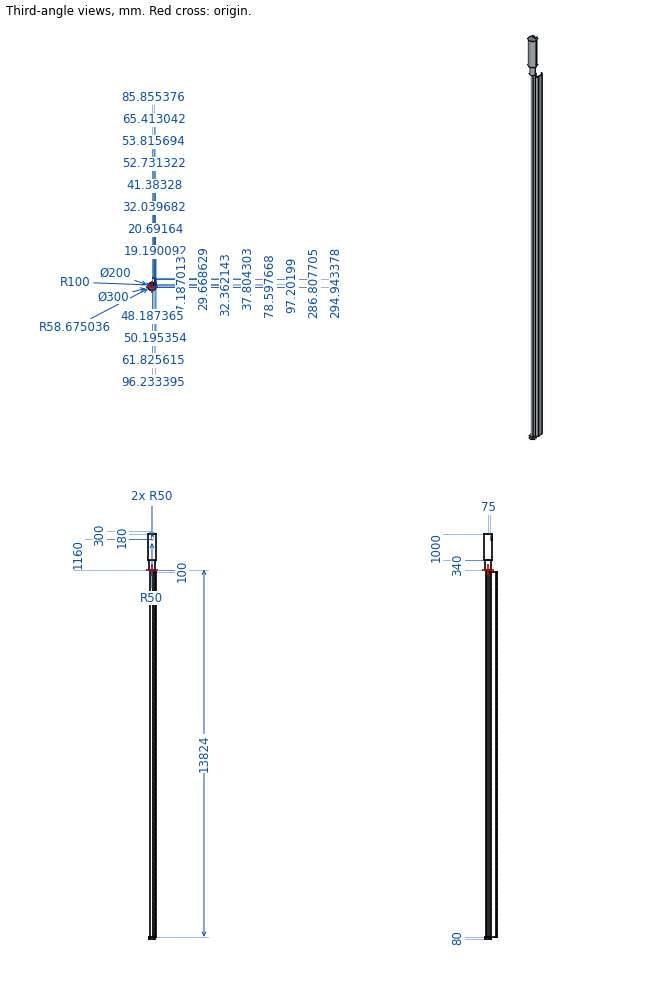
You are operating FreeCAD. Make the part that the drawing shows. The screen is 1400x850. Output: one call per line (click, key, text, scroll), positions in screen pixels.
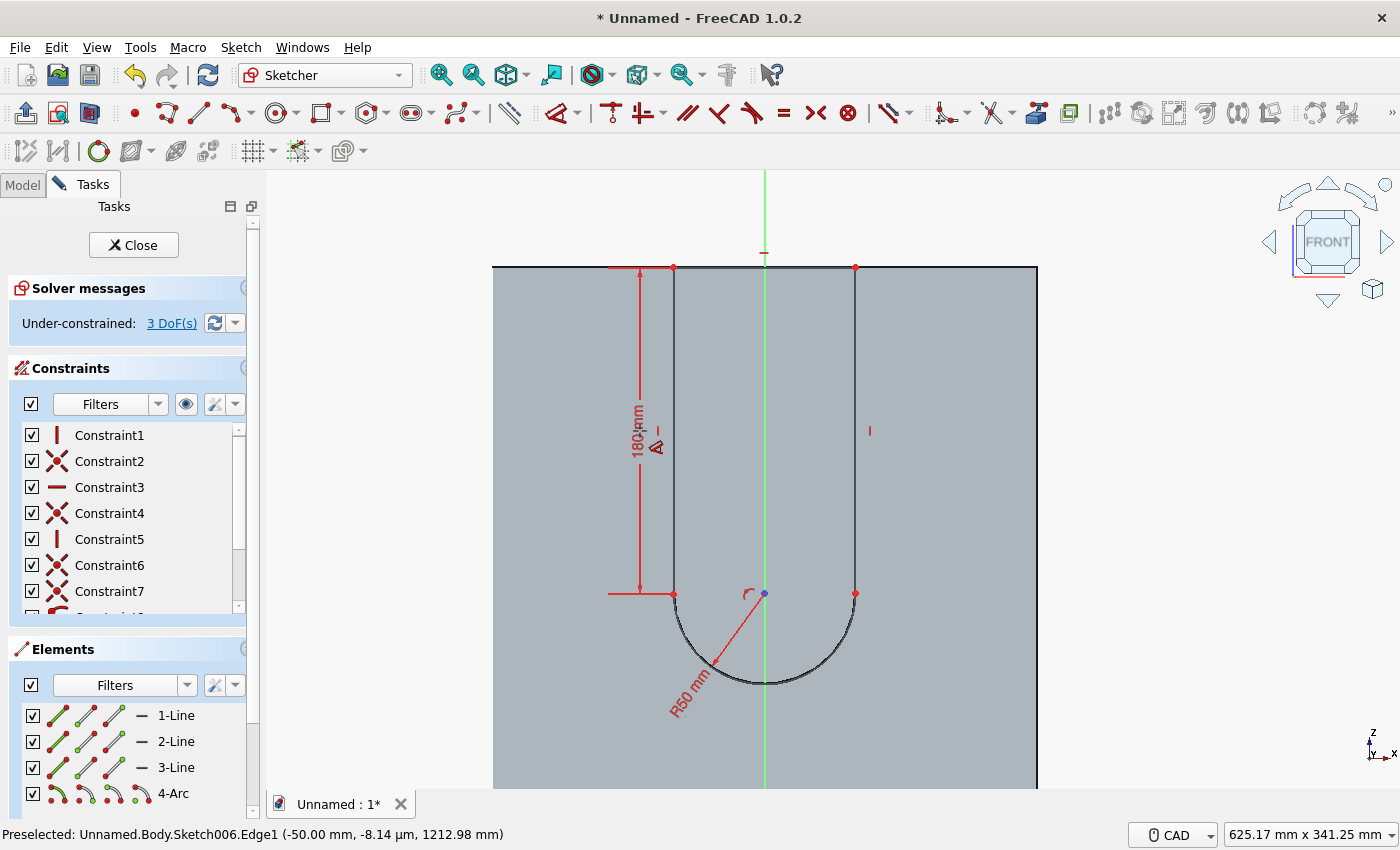
click(855, 366)
click(889, 431)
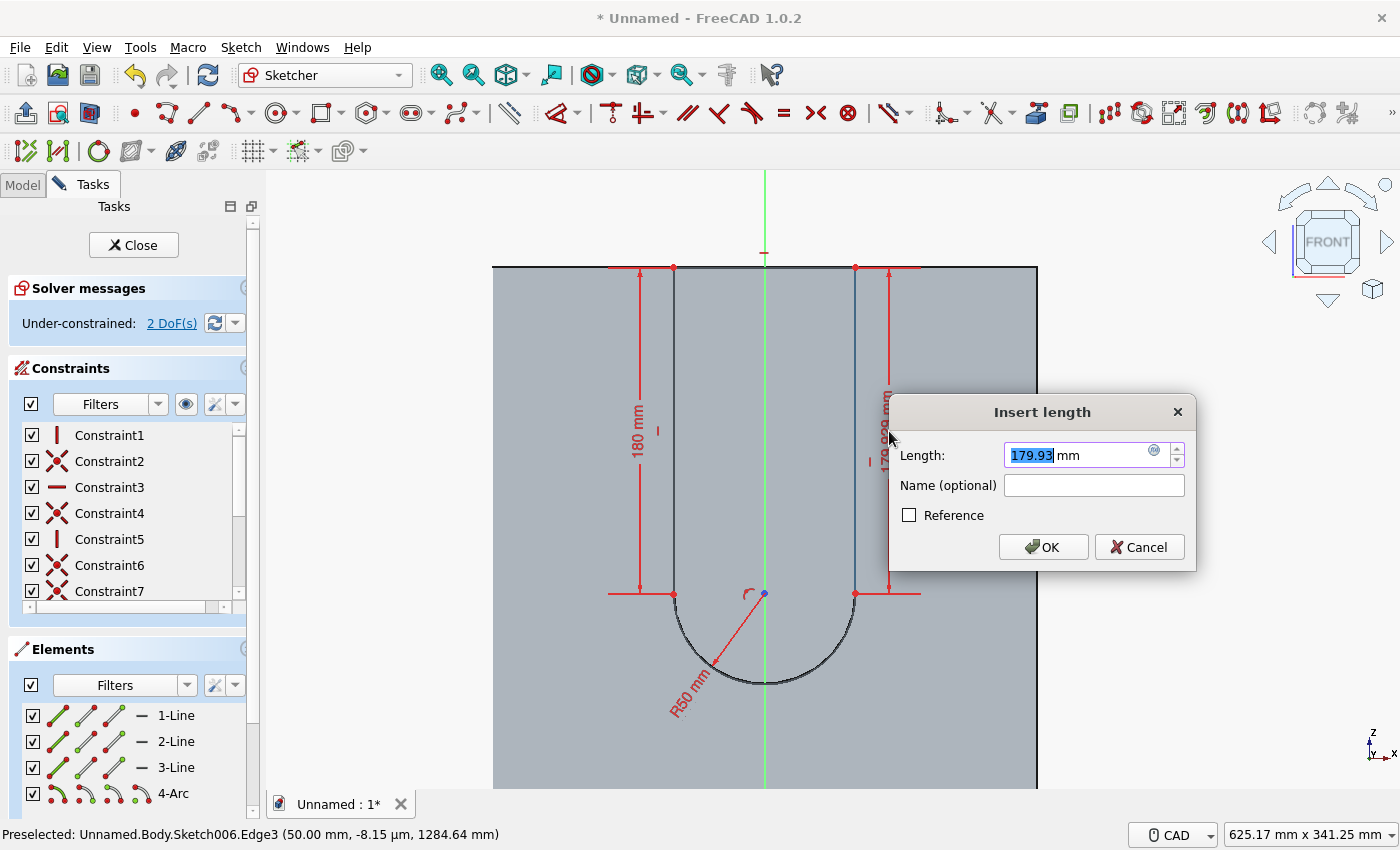
text(180)
key(Return)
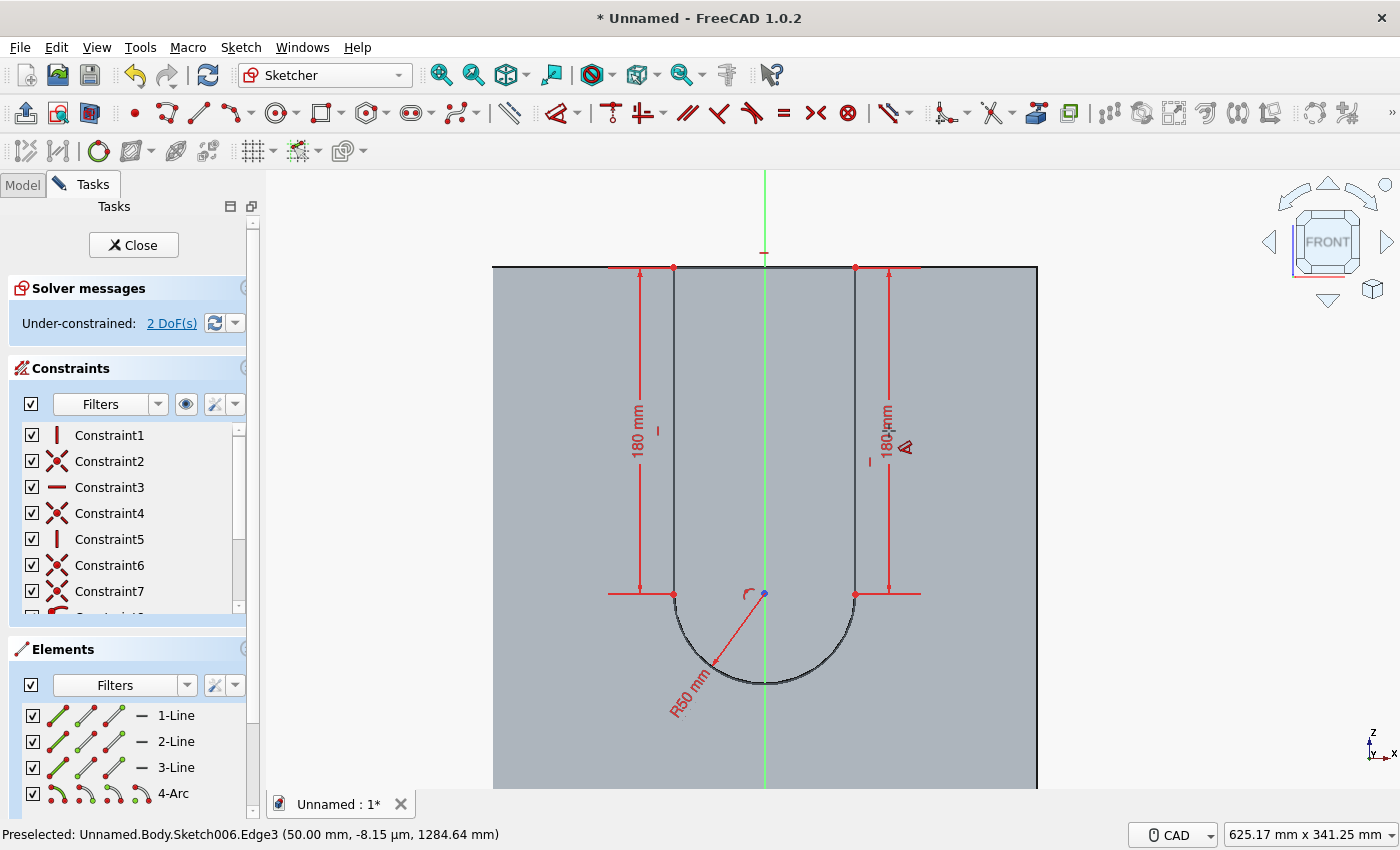
click(674, 594)
click(640, 639)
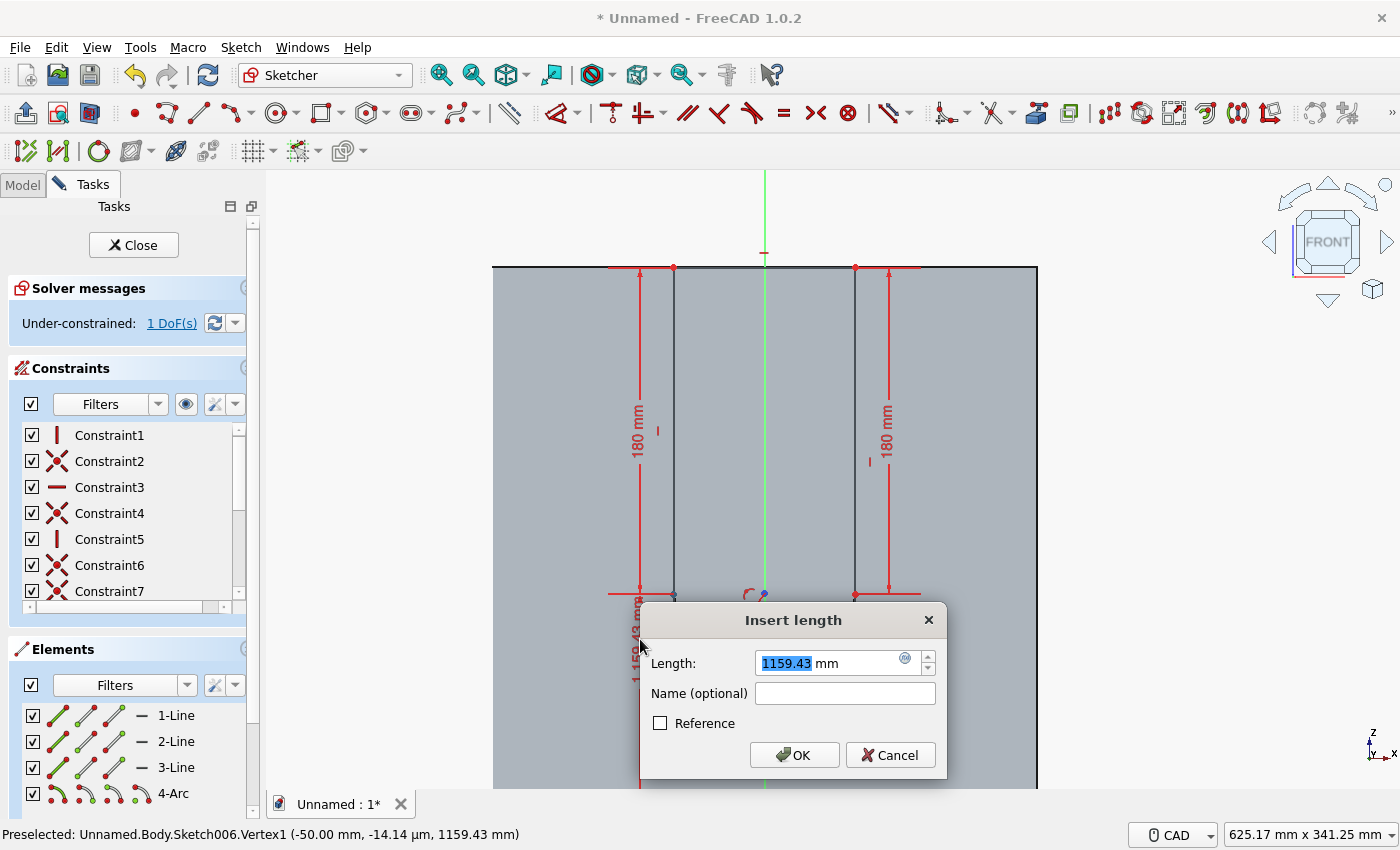
text(1160)
key(Return)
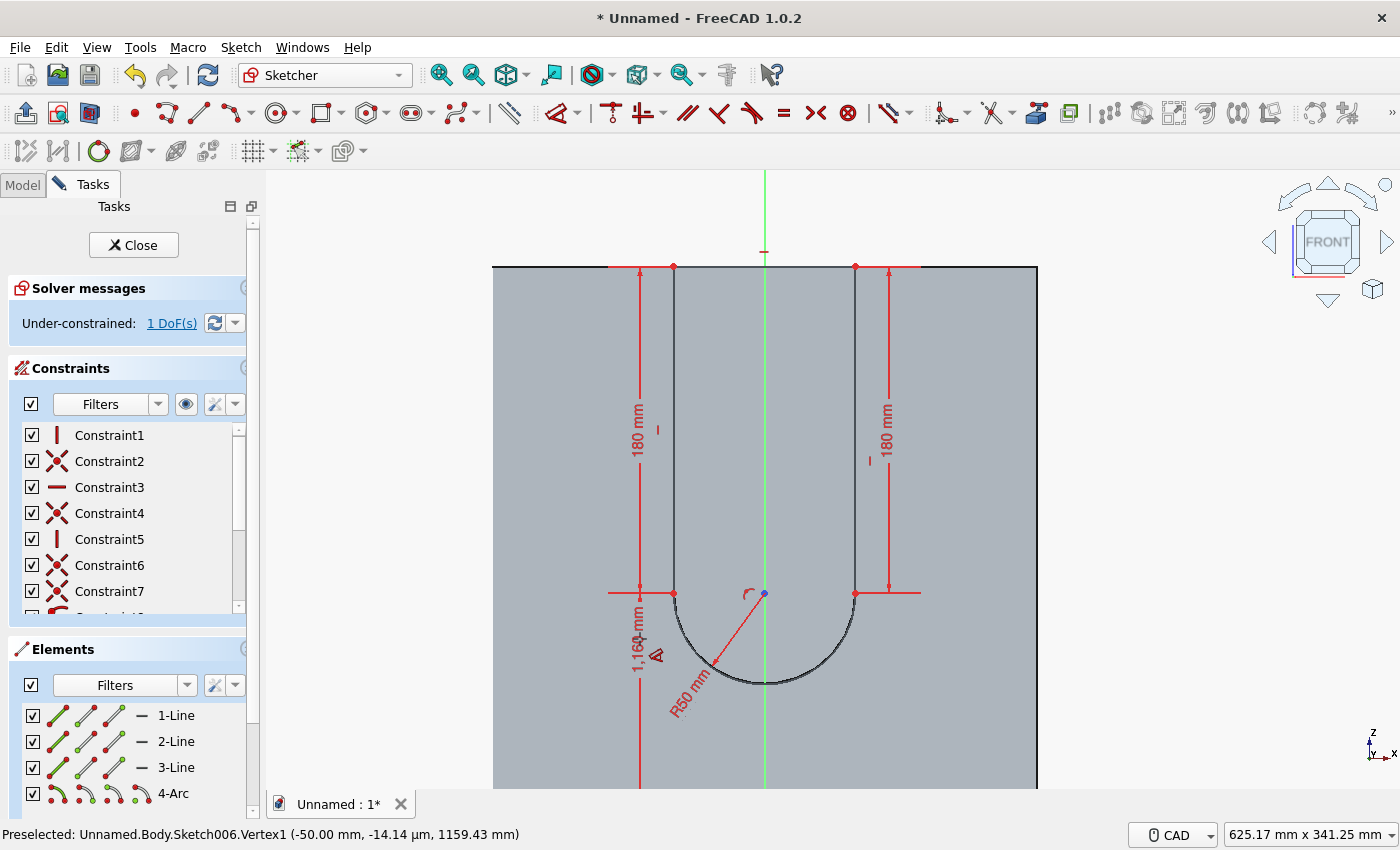
click(765, 594)
click(799, 639)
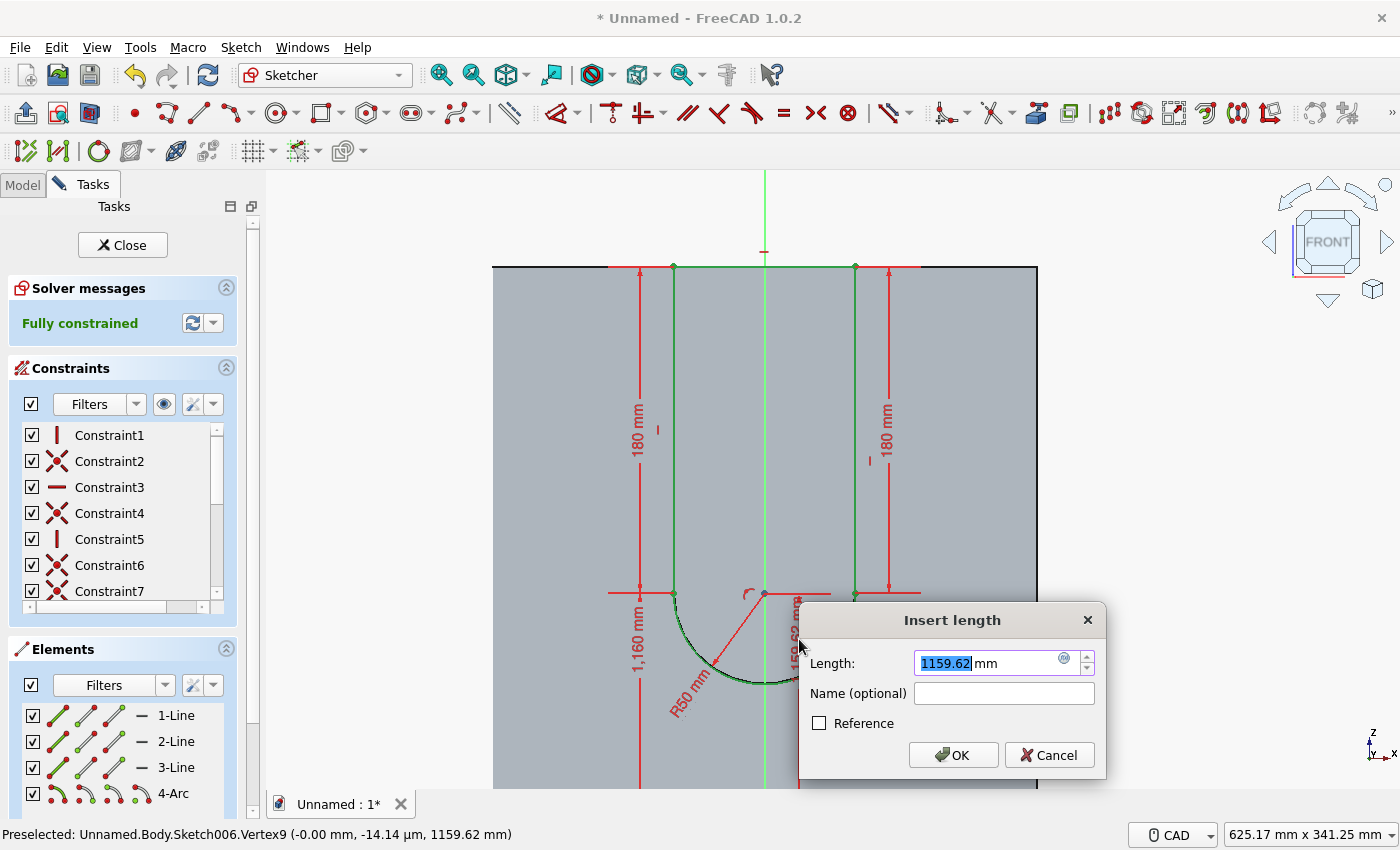
text(1160)
key(Return)
key(Escape)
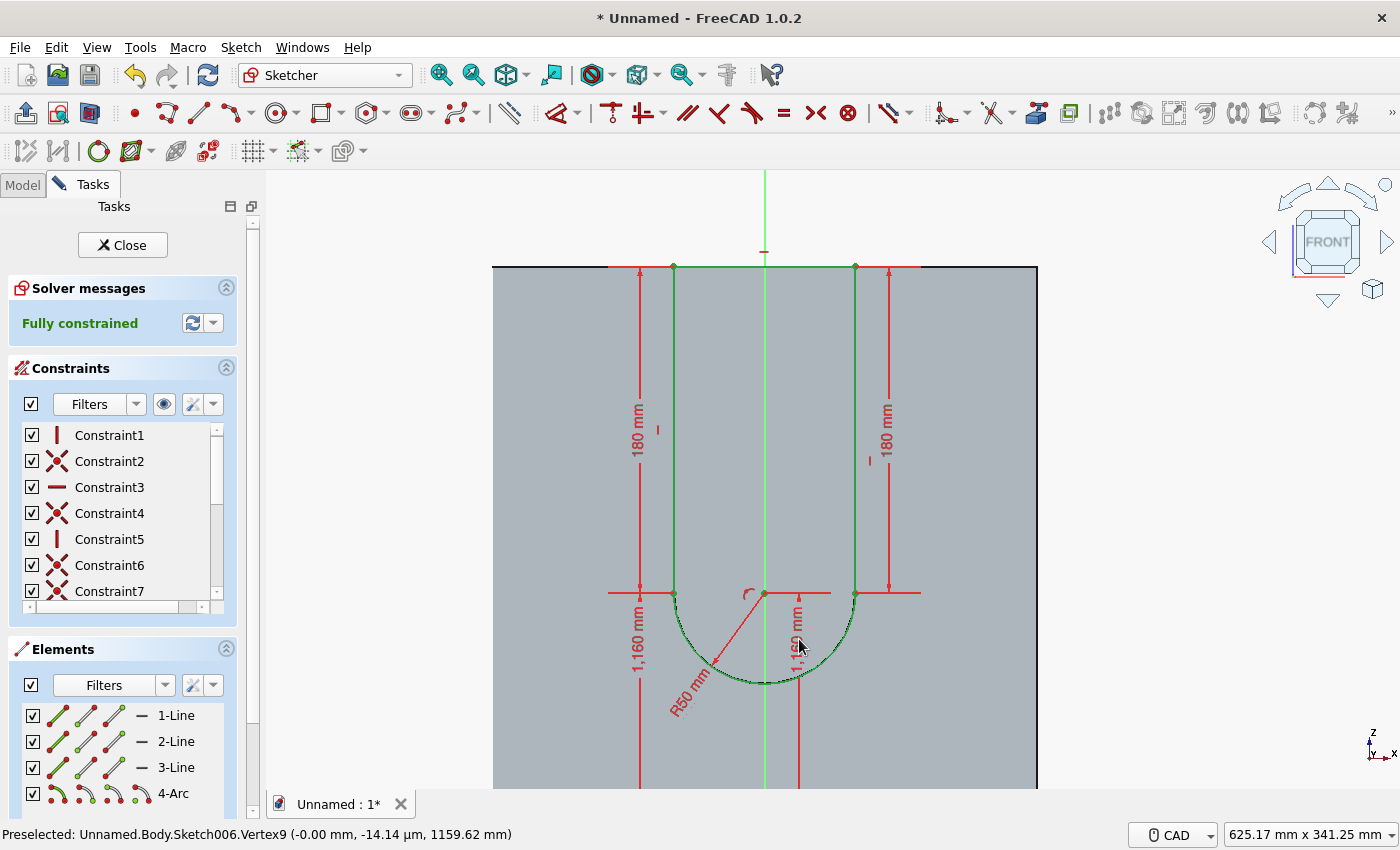
click(123, 245)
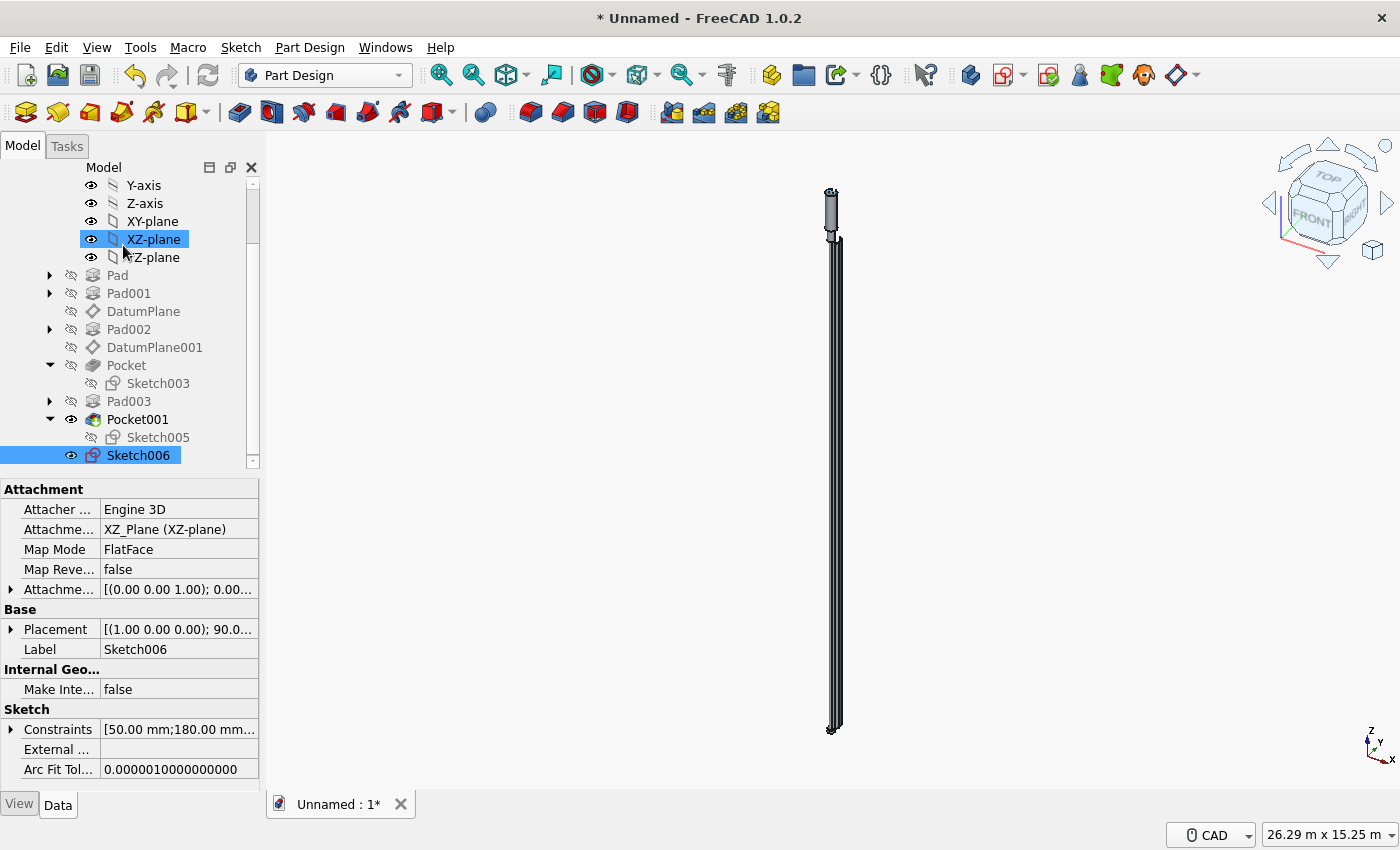
click(26, 112)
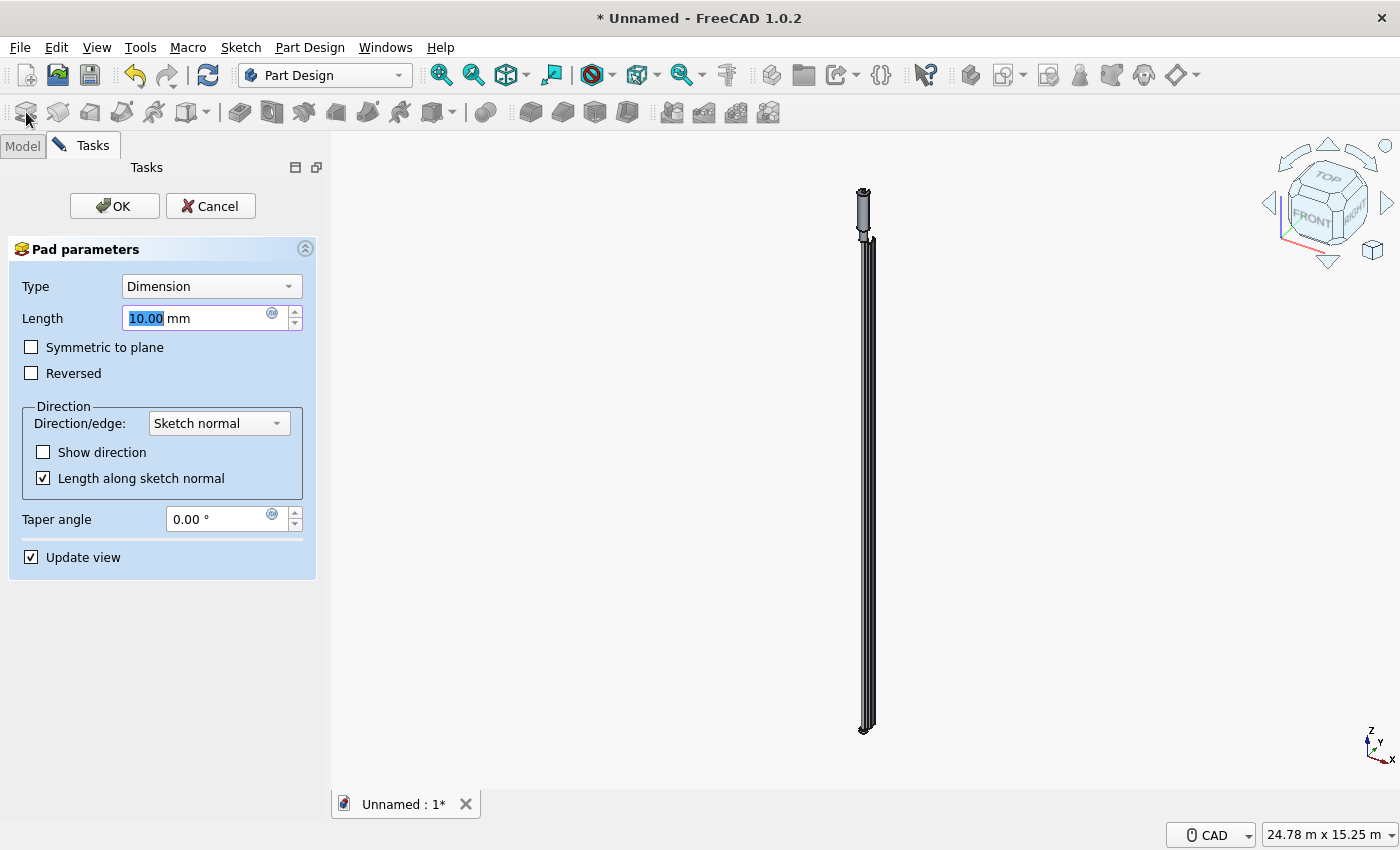
text(75)
key(Tab)